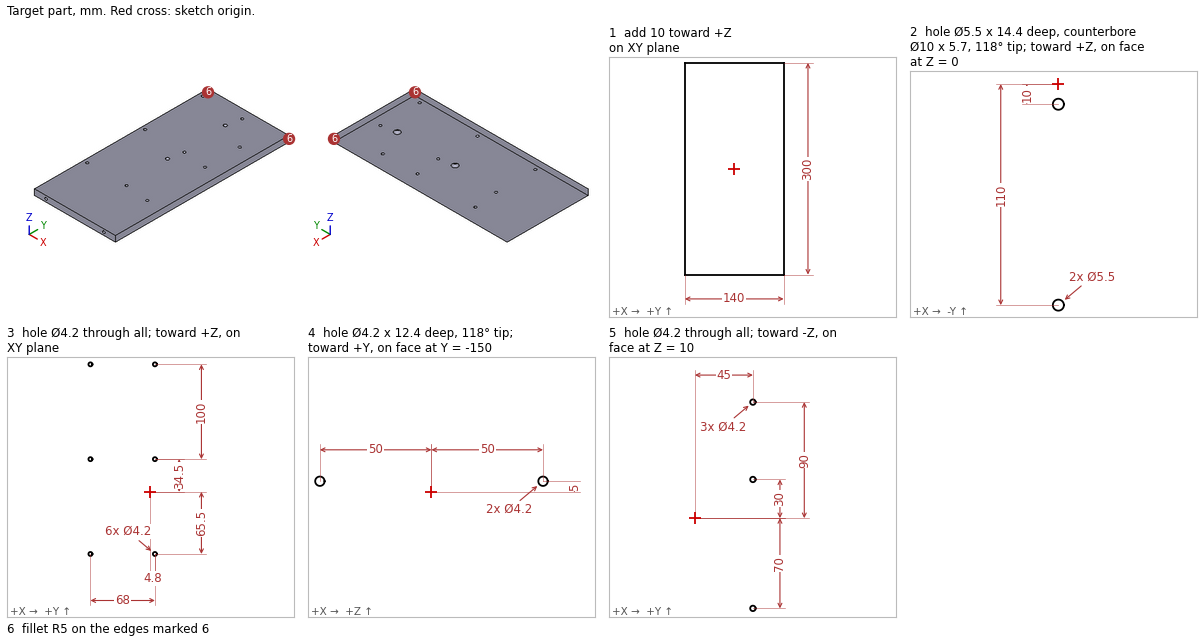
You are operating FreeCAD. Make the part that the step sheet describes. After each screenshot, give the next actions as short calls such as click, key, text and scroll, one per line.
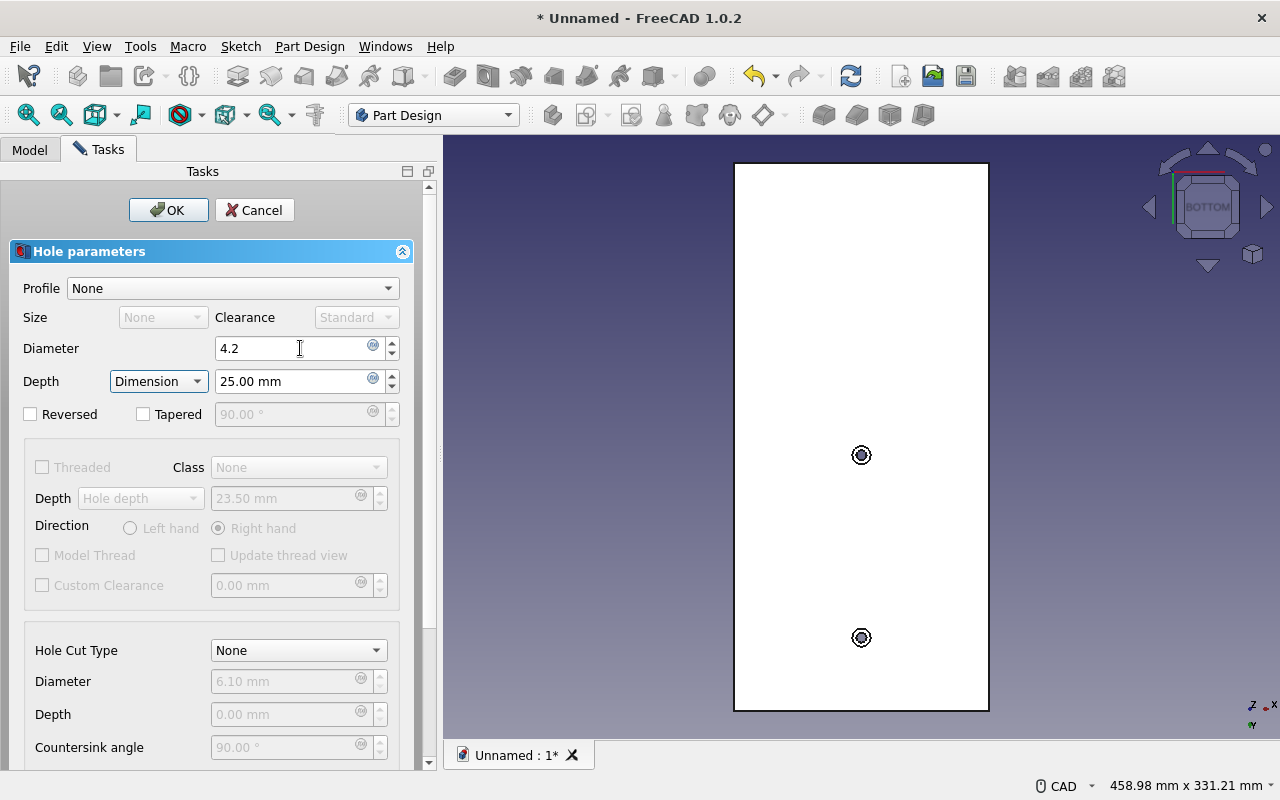
click(160, 382)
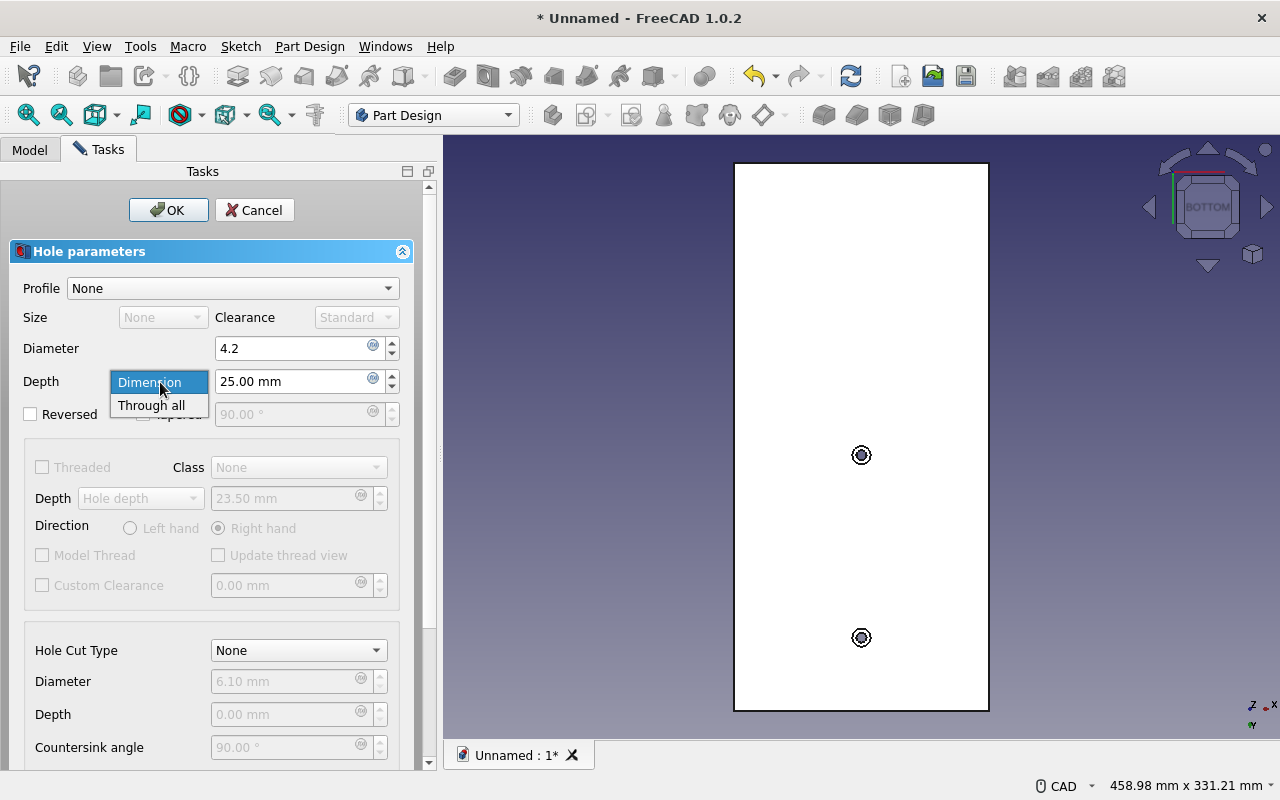
click(158, 406)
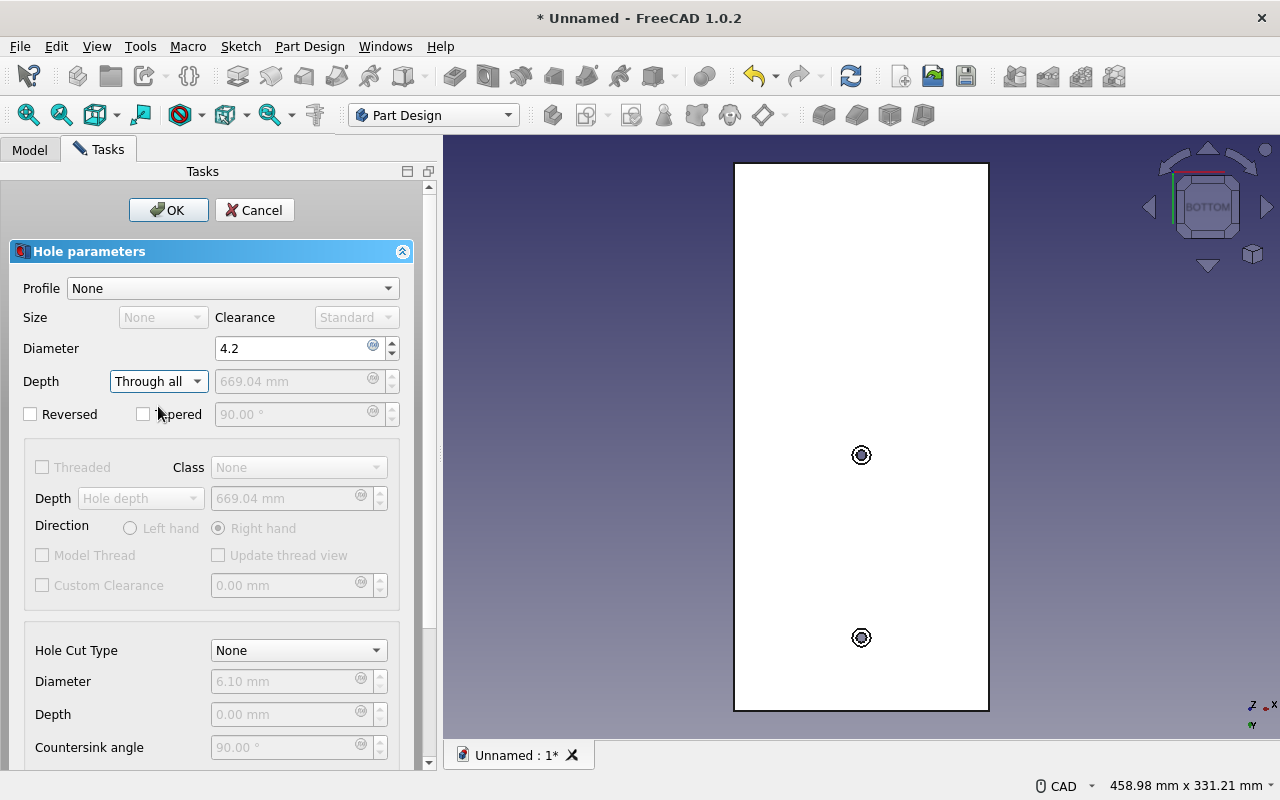
click(31, 414)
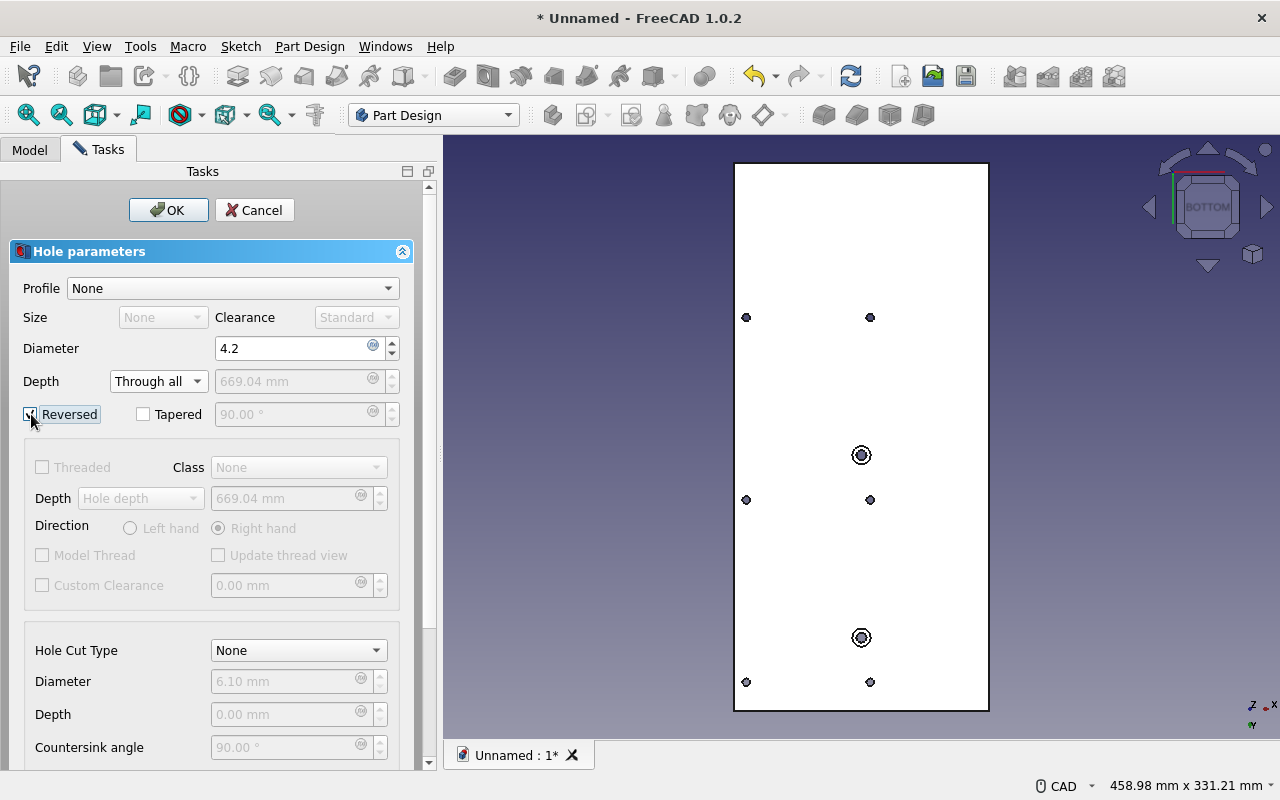
click(169, 210)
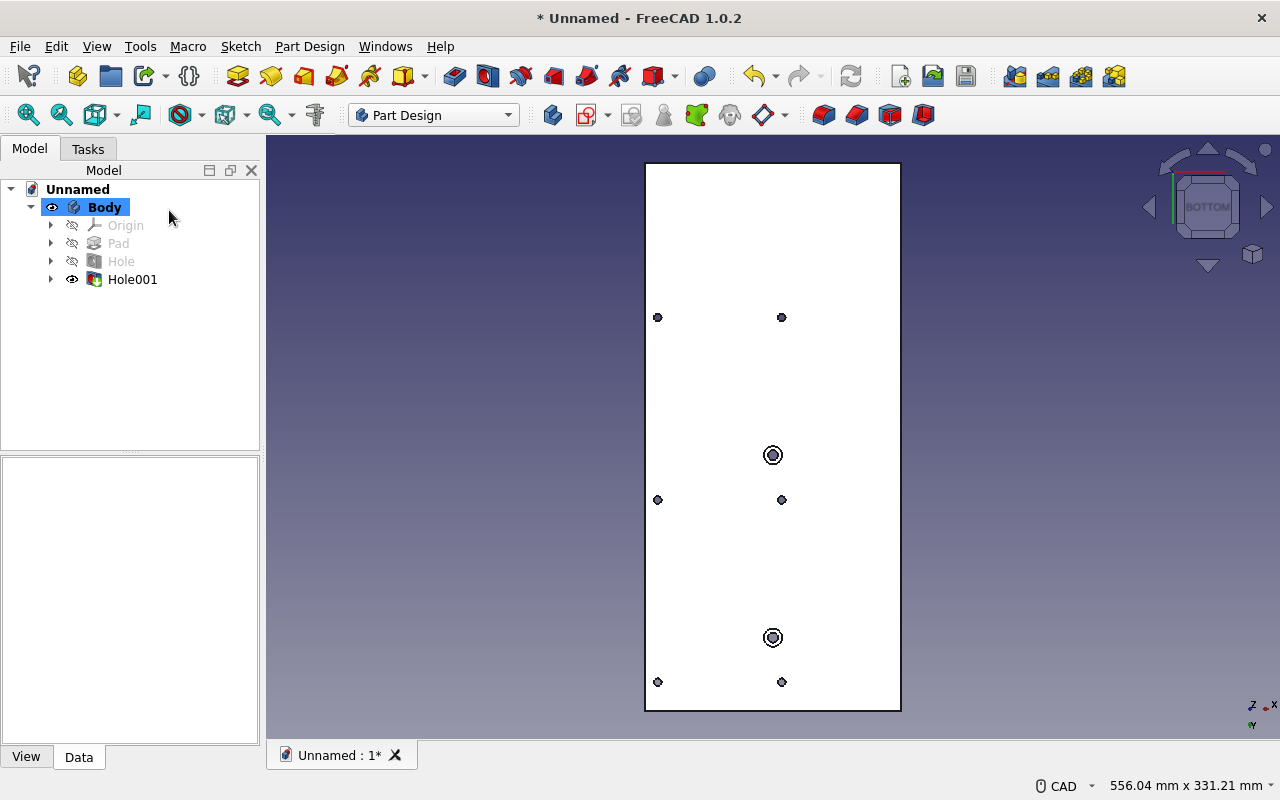
key(0)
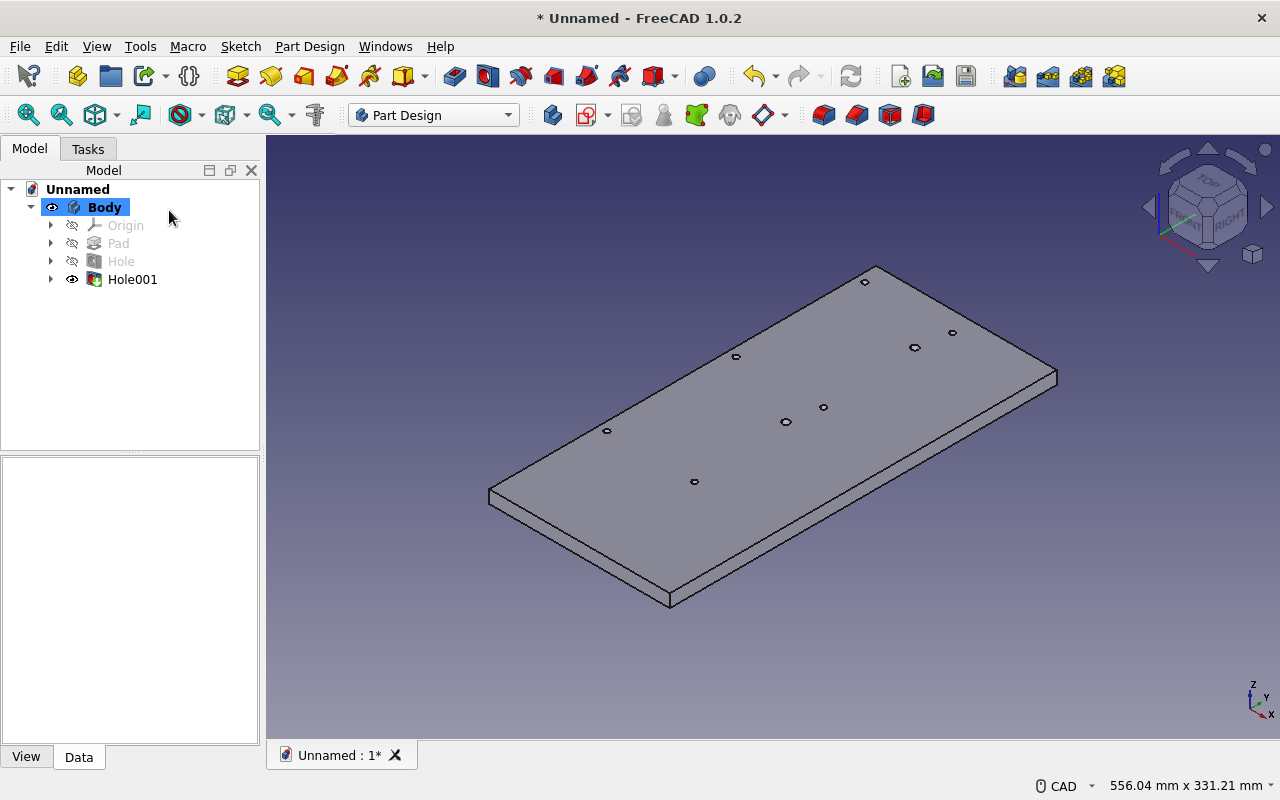
key(1)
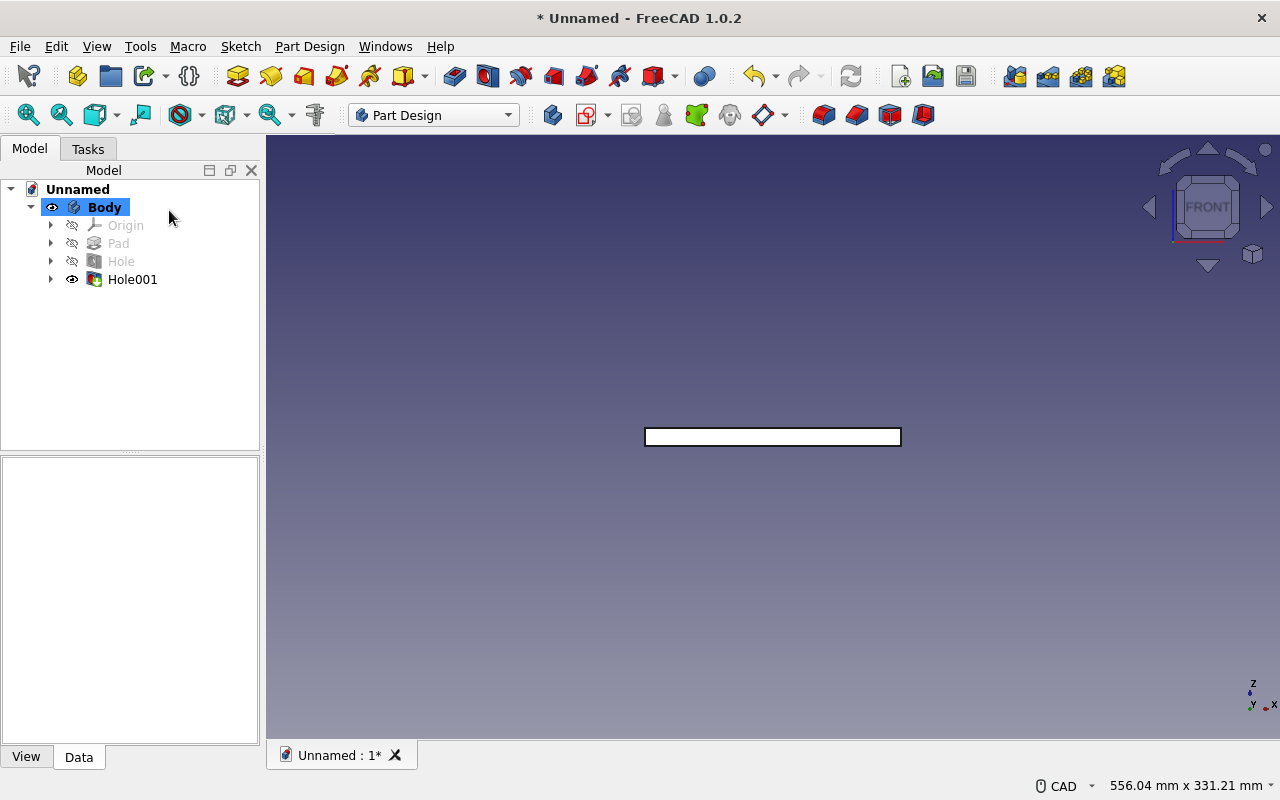
click(29, 116)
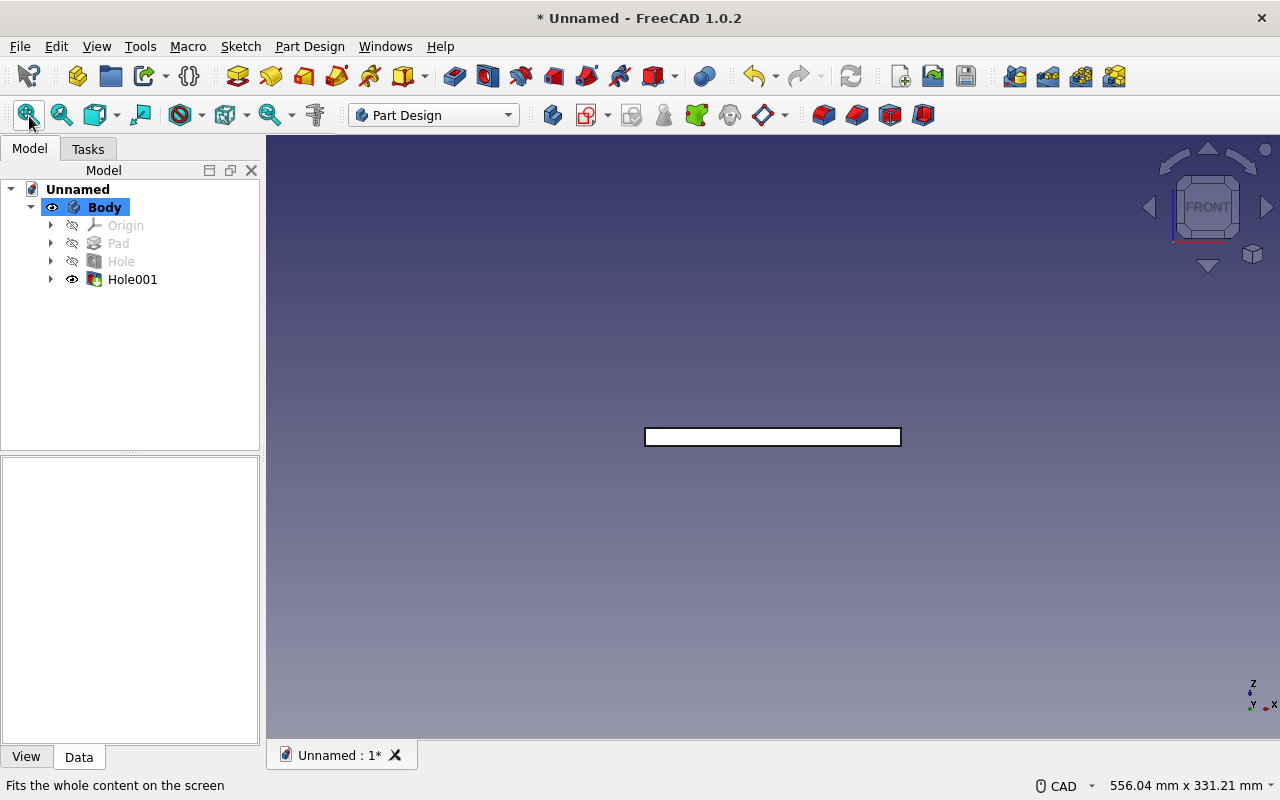
click(882, 436)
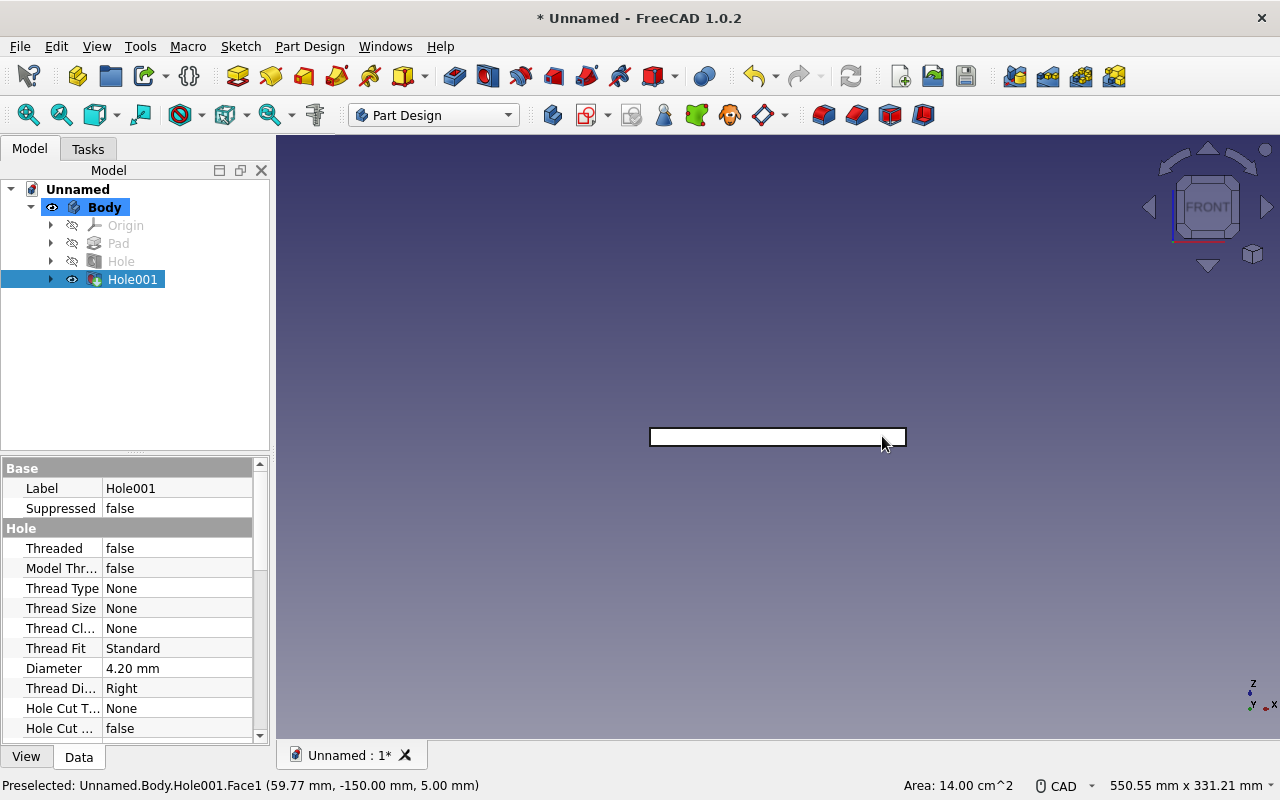
click(586, 116)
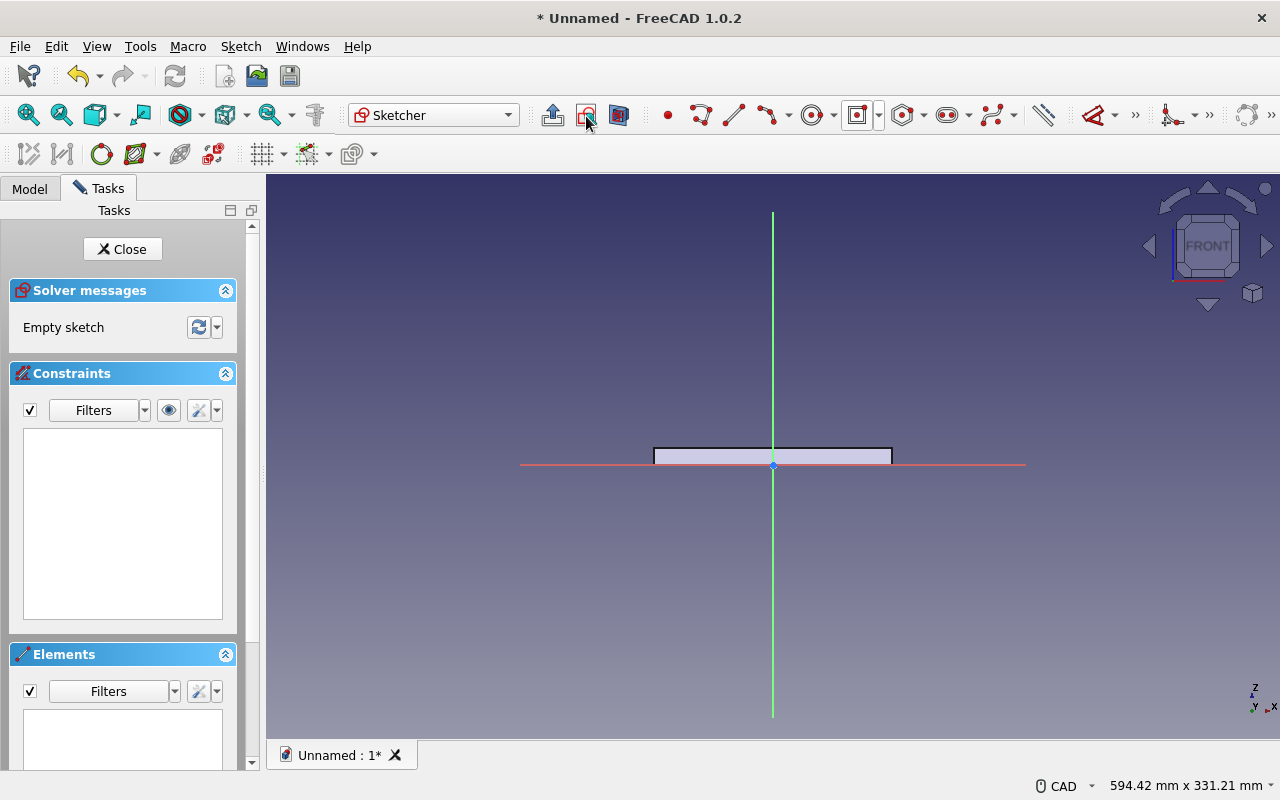
scroll(803, 460, up, 6)